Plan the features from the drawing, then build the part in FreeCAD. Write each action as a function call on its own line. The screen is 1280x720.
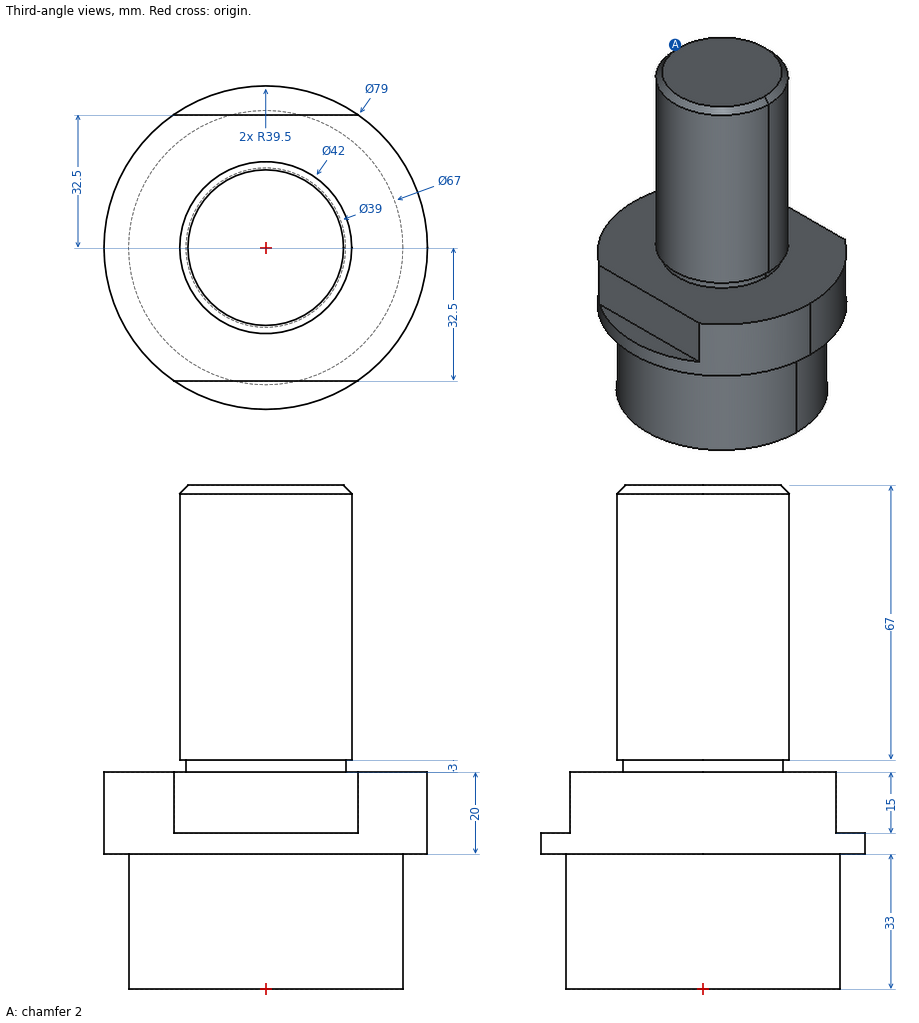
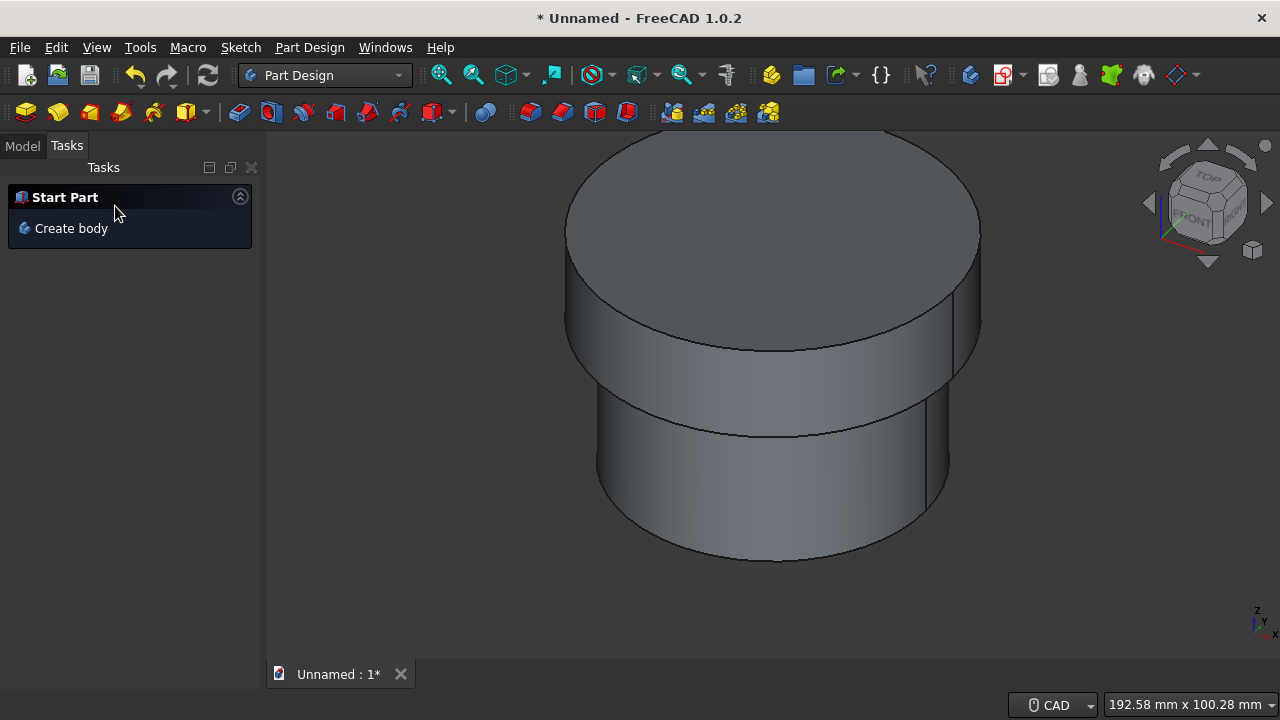
click(442, 76)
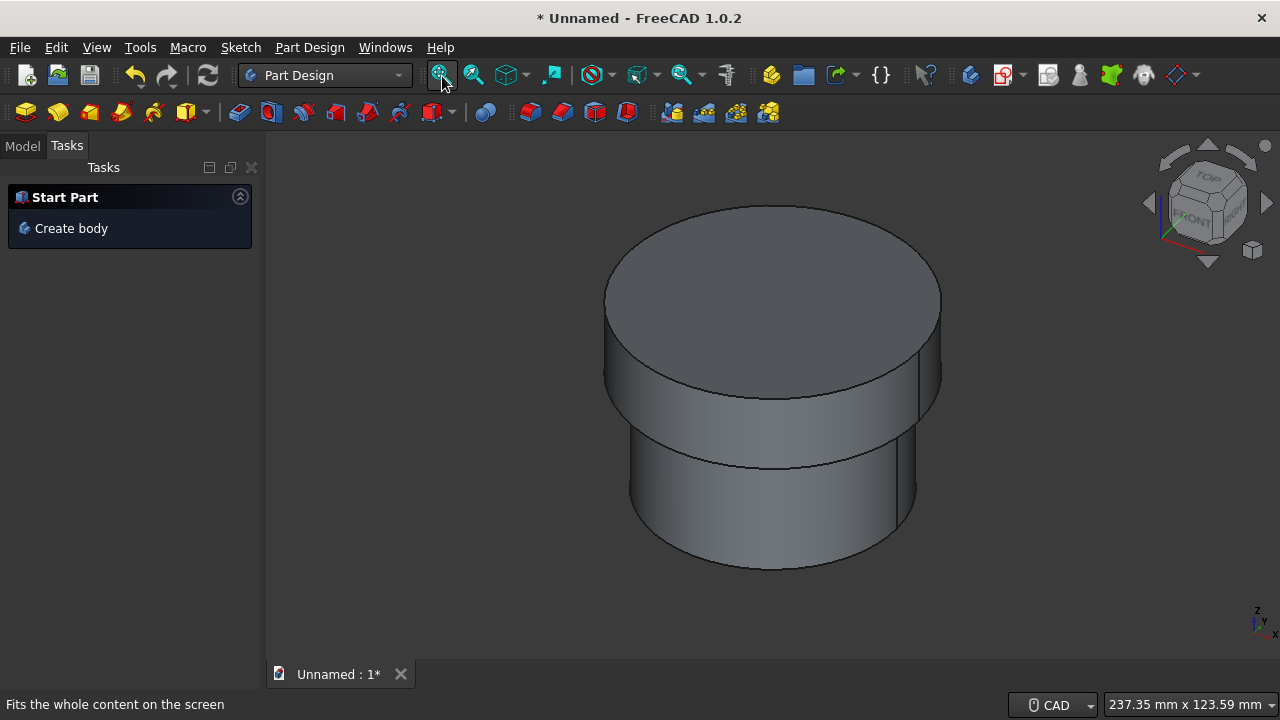
click(23, 145)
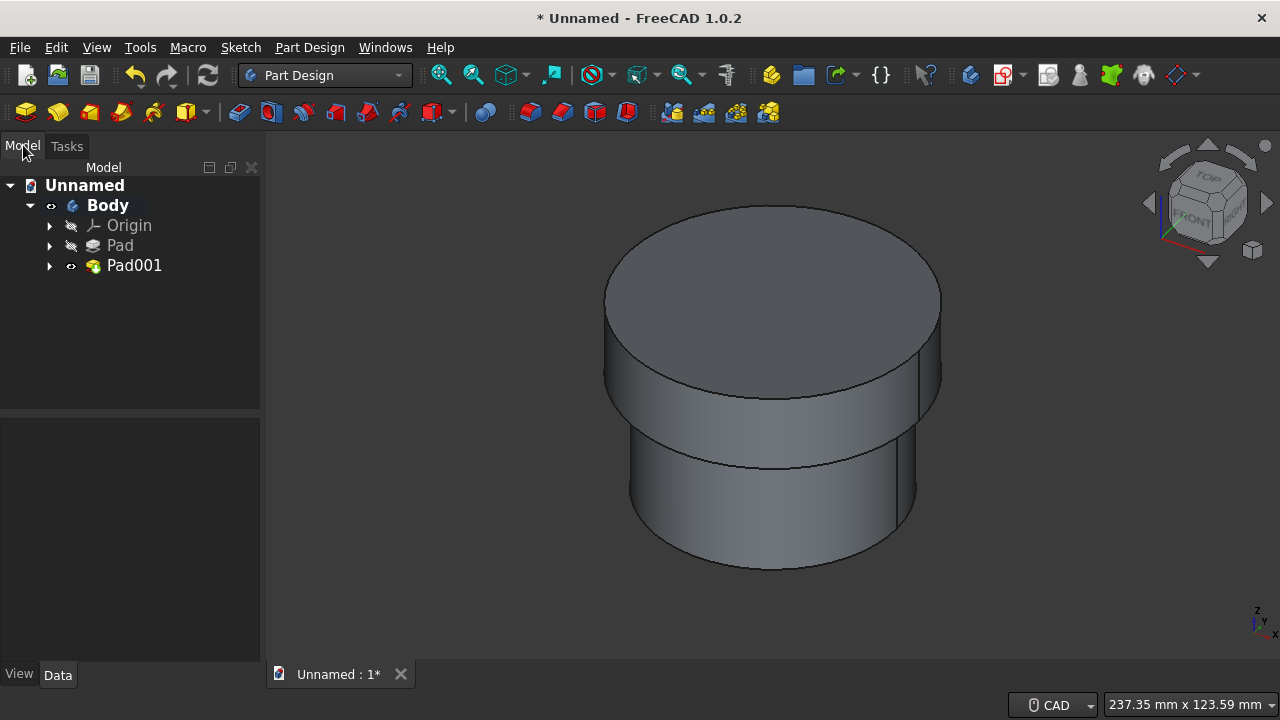
click(50, 226)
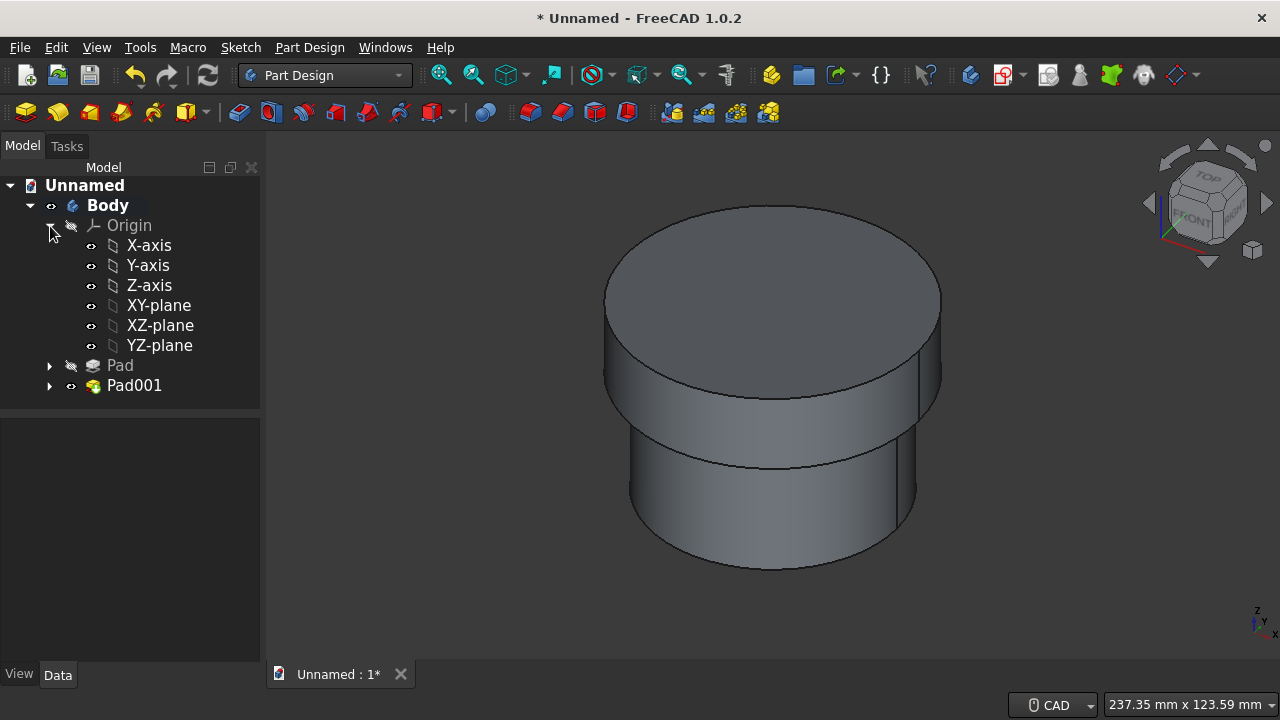
click(136, 306)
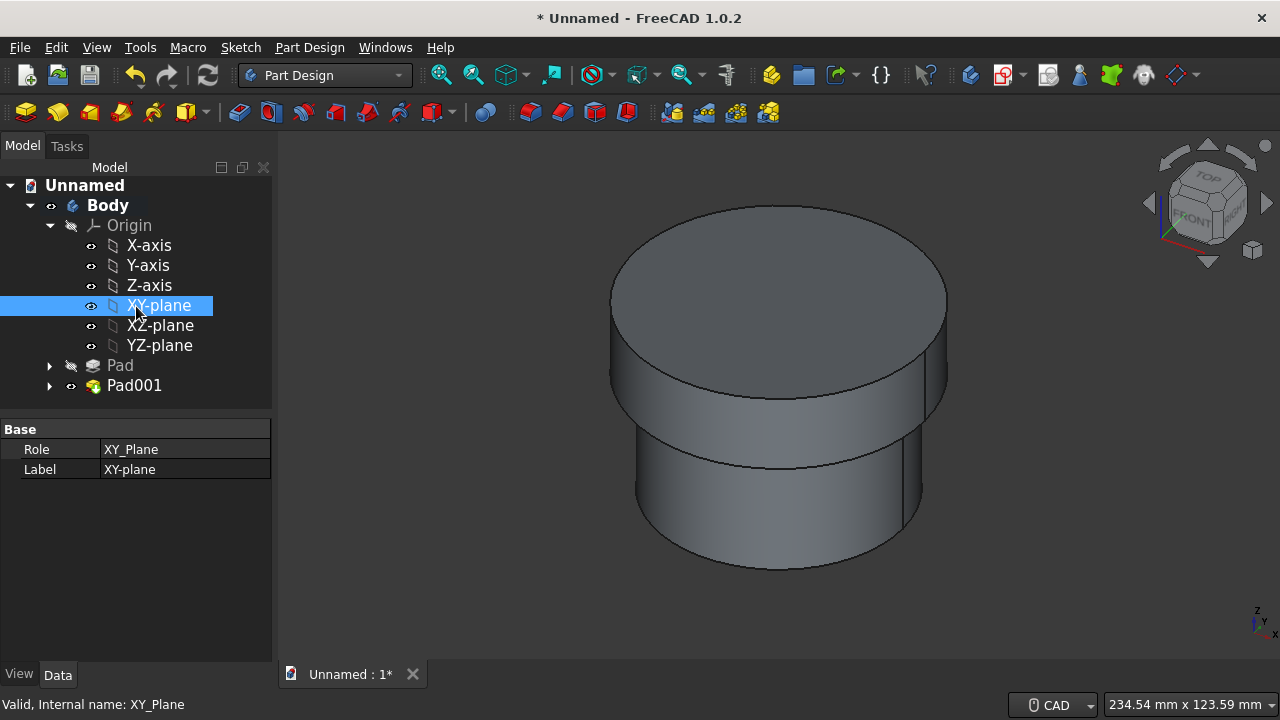
click(1176, 76)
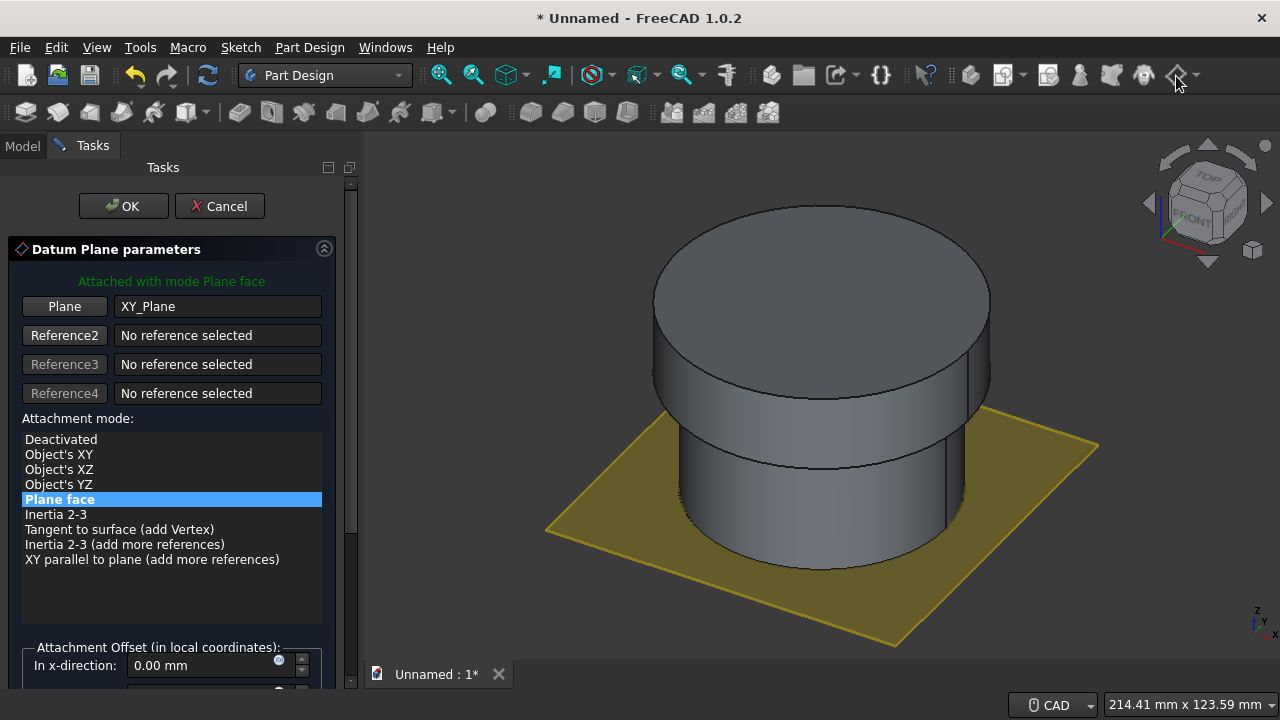
scroll(351, 432, down, 2)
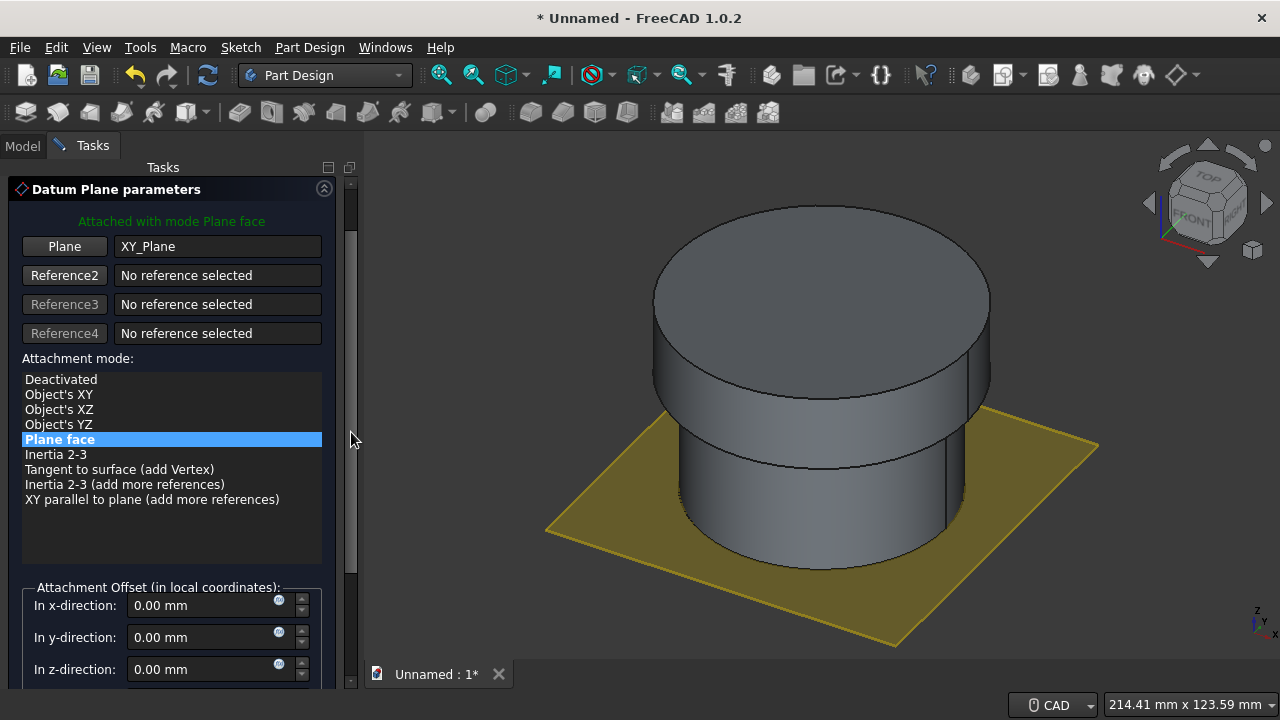
triple_click(210, 609)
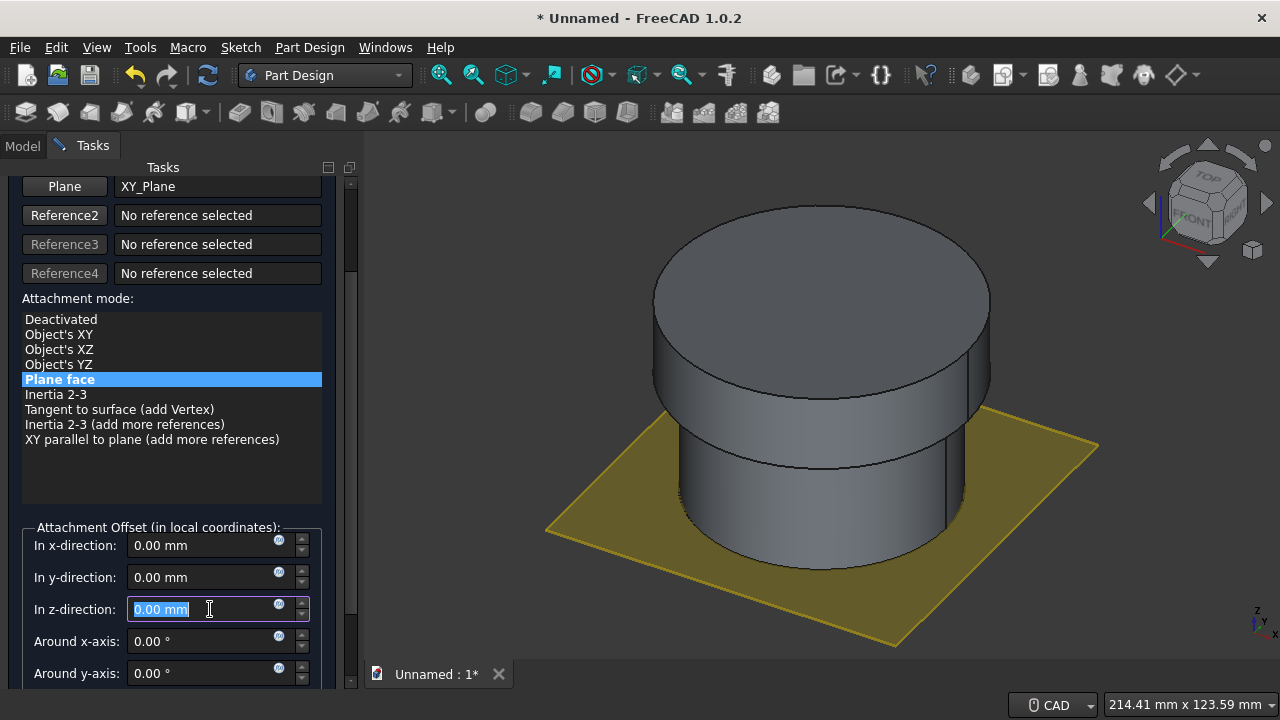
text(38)
key(Tab)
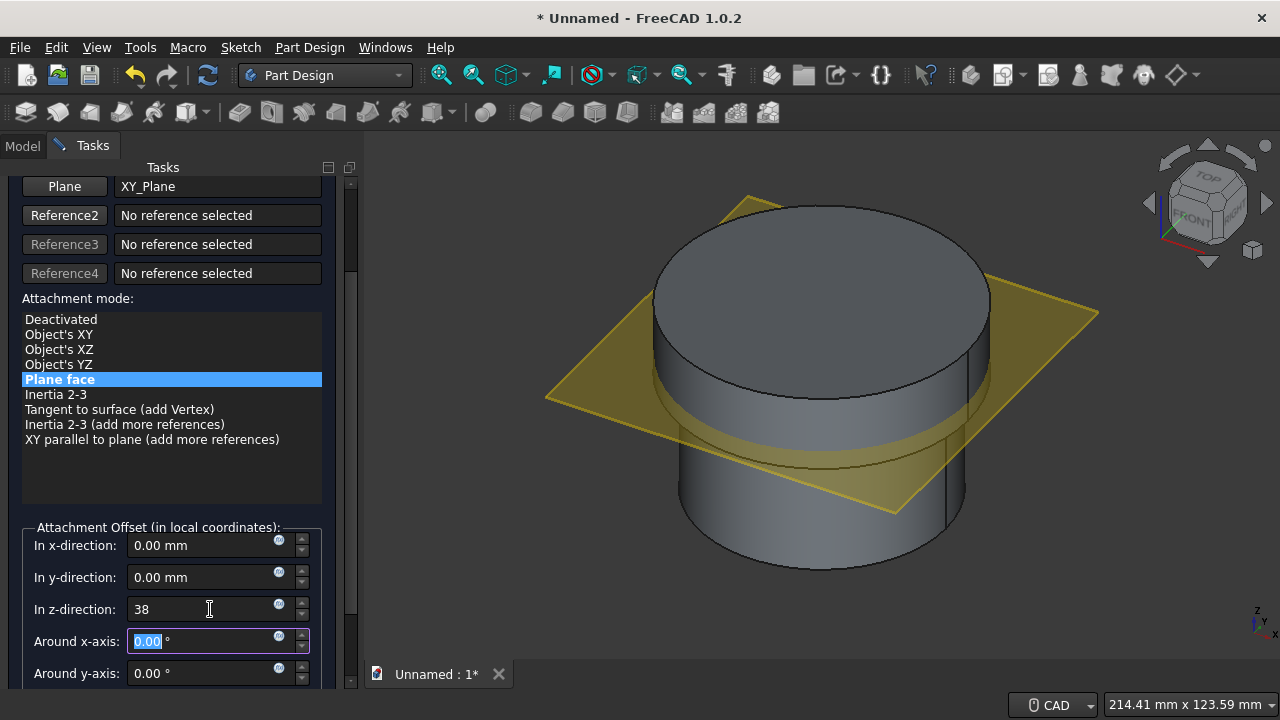
scroll(351, 432, up, 3)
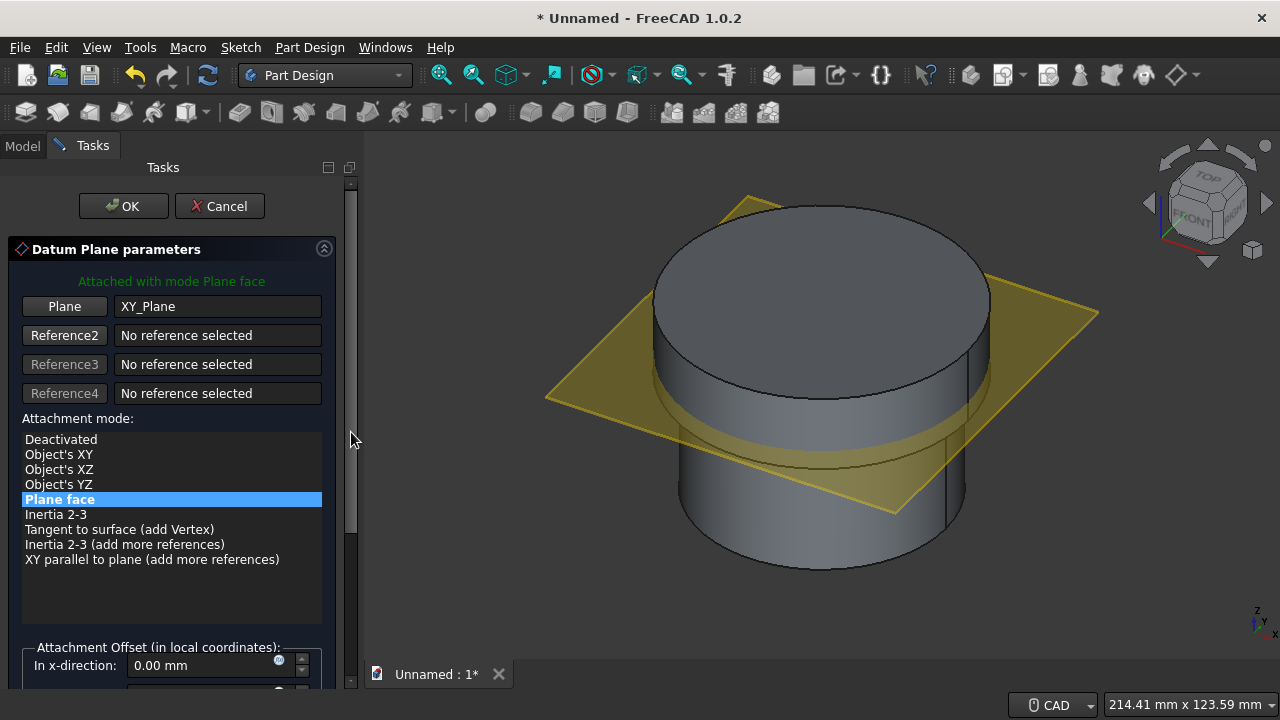
click(124, 206)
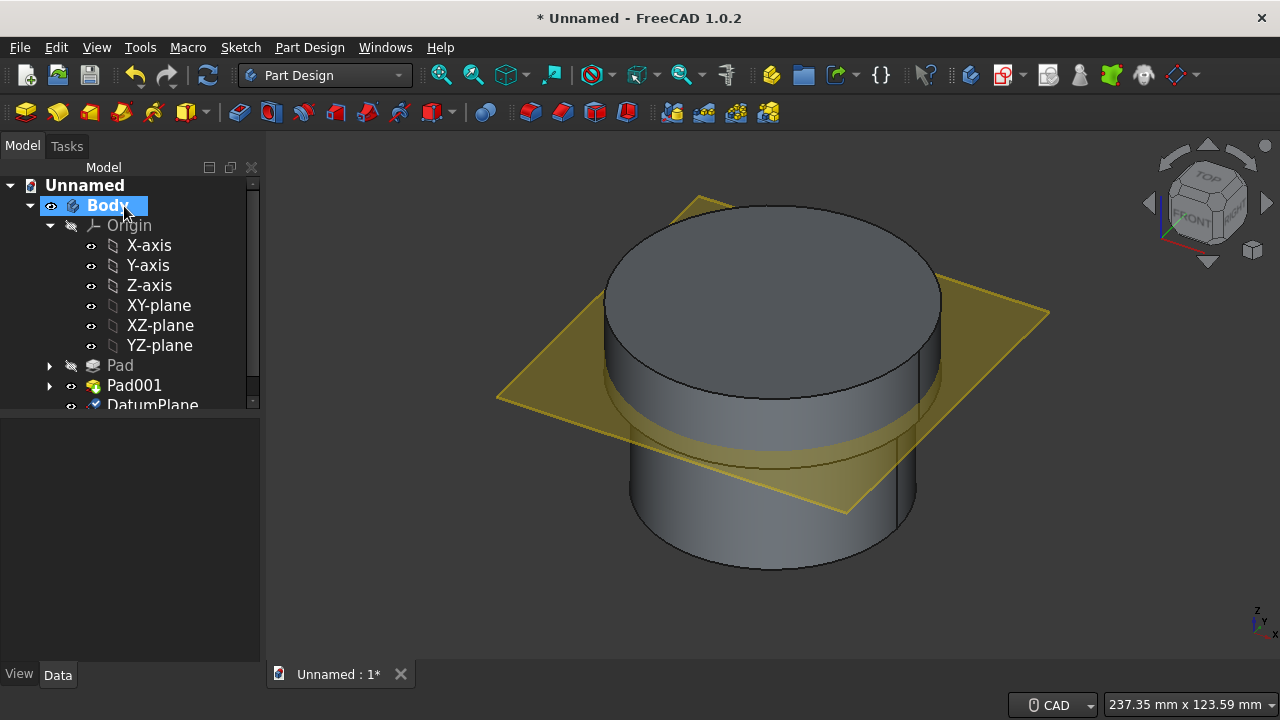
click(116, 406)